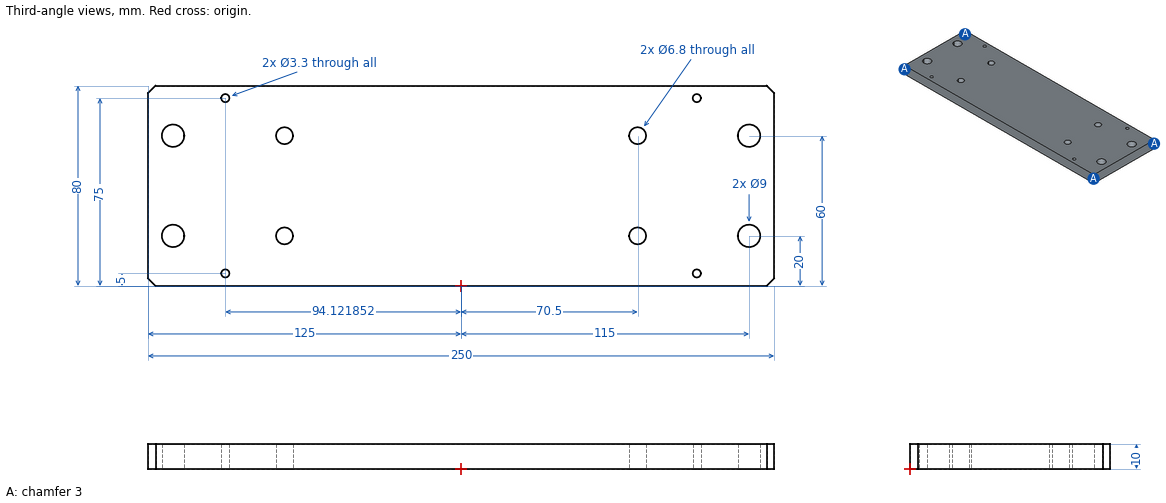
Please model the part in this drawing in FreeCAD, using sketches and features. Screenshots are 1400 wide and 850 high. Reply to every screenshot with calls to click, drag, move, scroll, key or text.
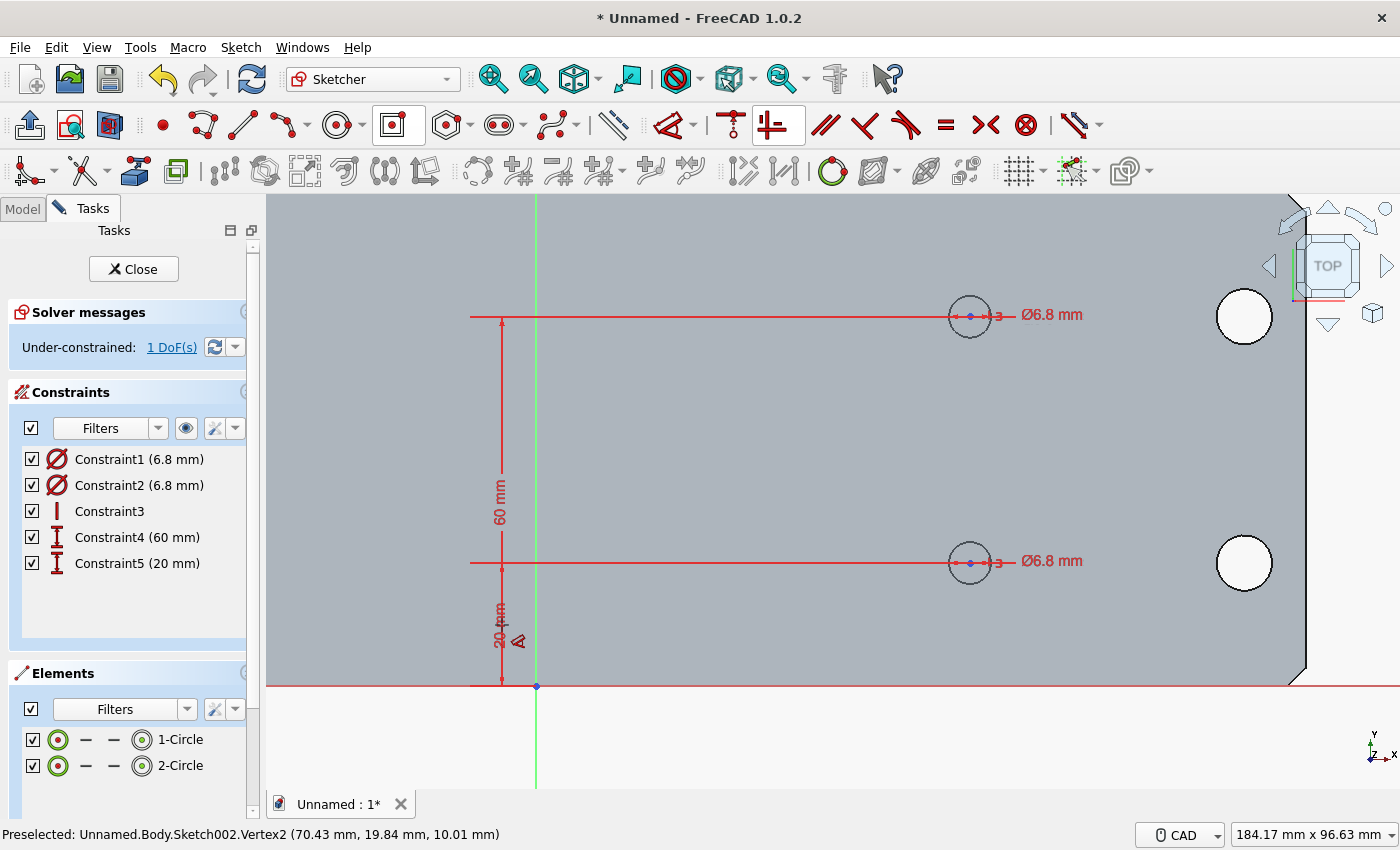
click(970, 317)
click(753, 720)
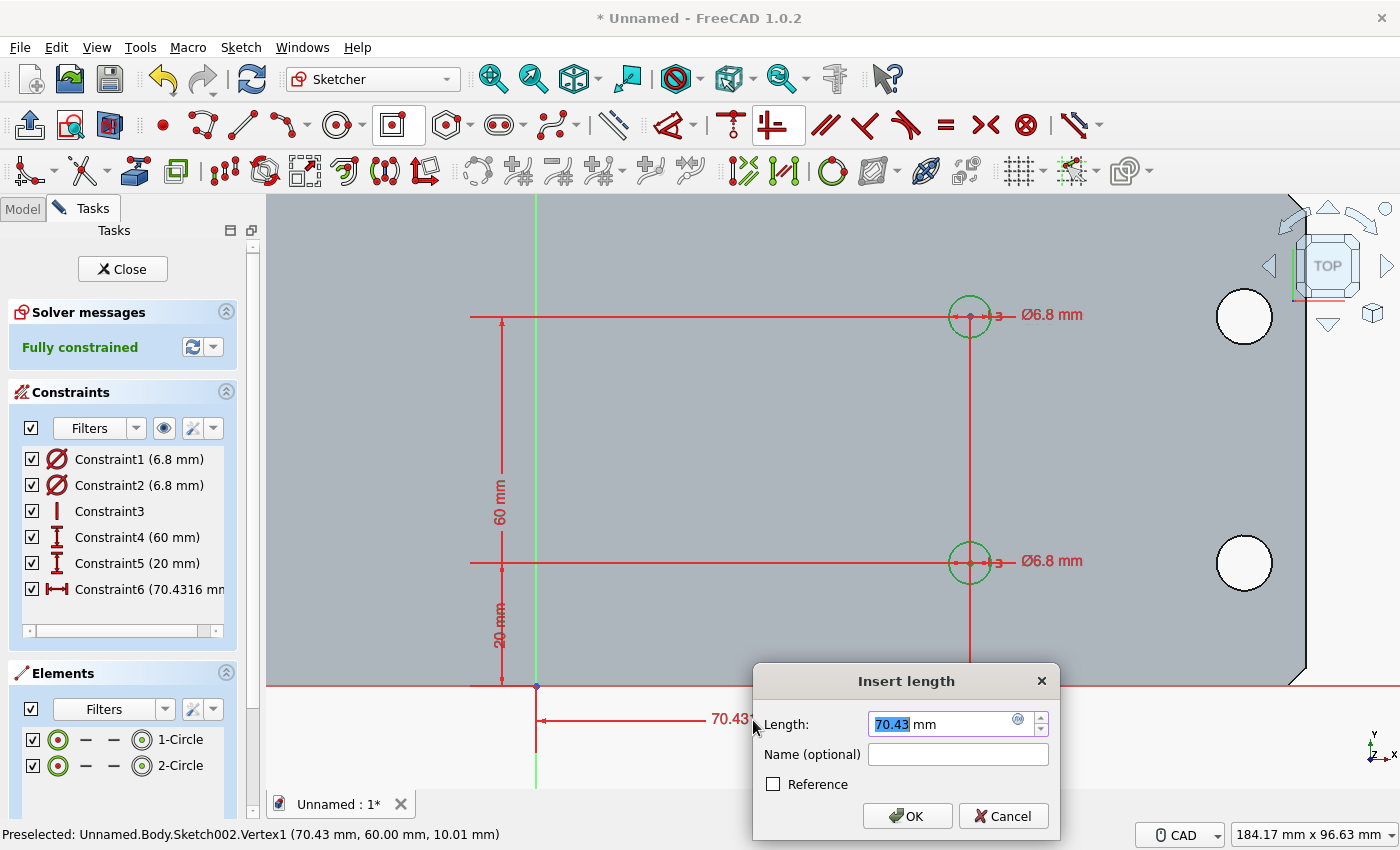
text(70.5)
key(Return)
key(Escape)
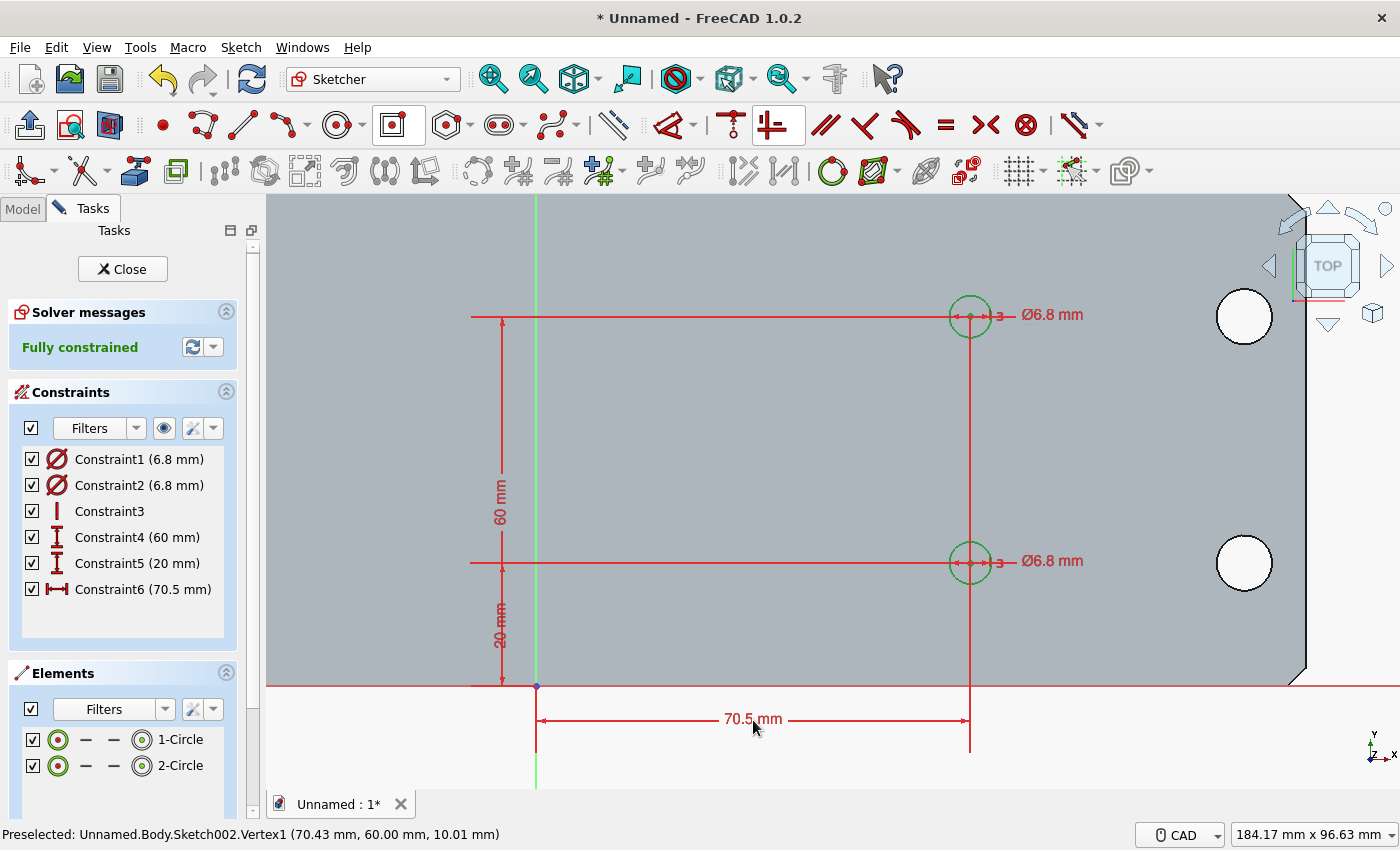
click(123, 269)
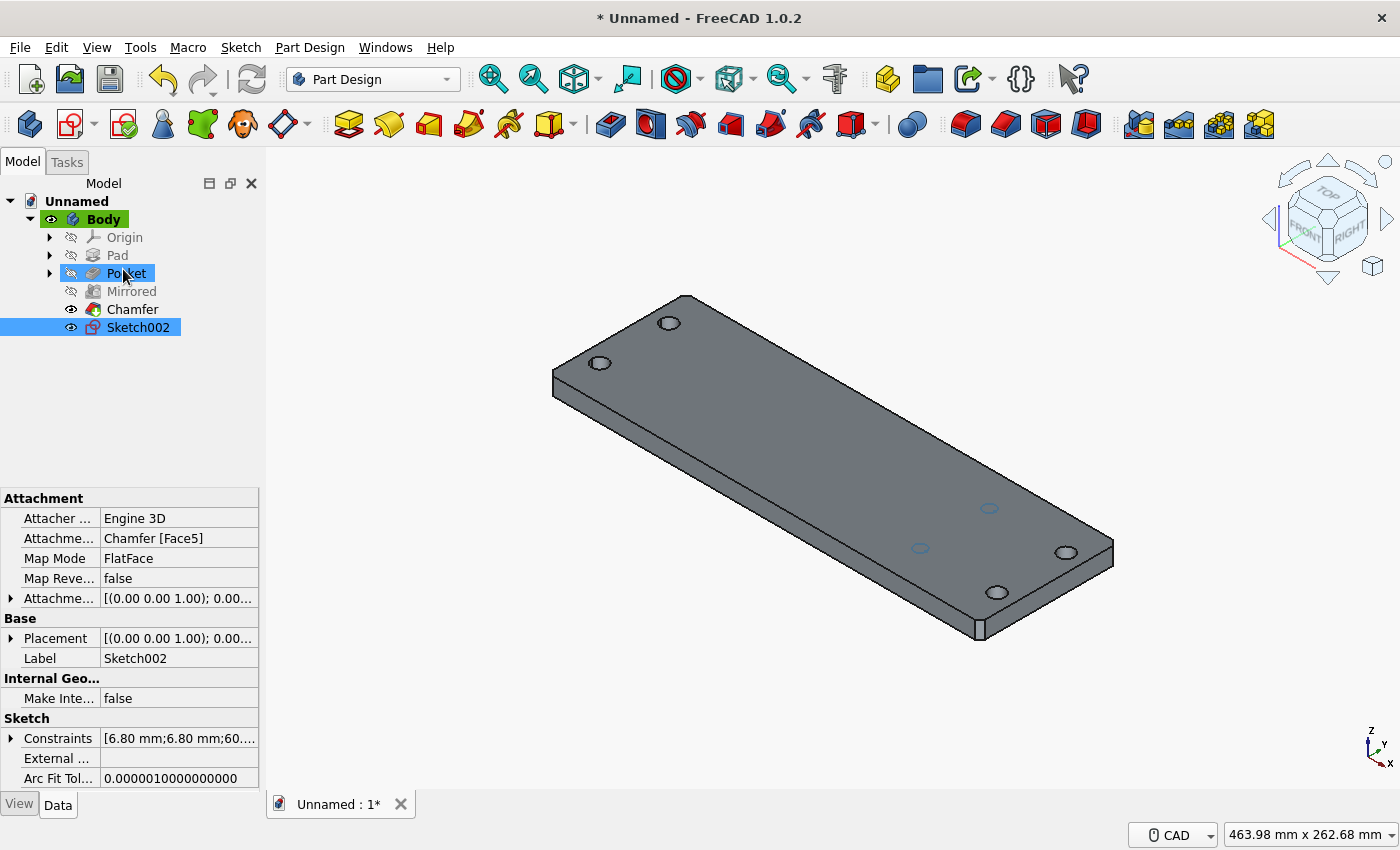
click(652, 124)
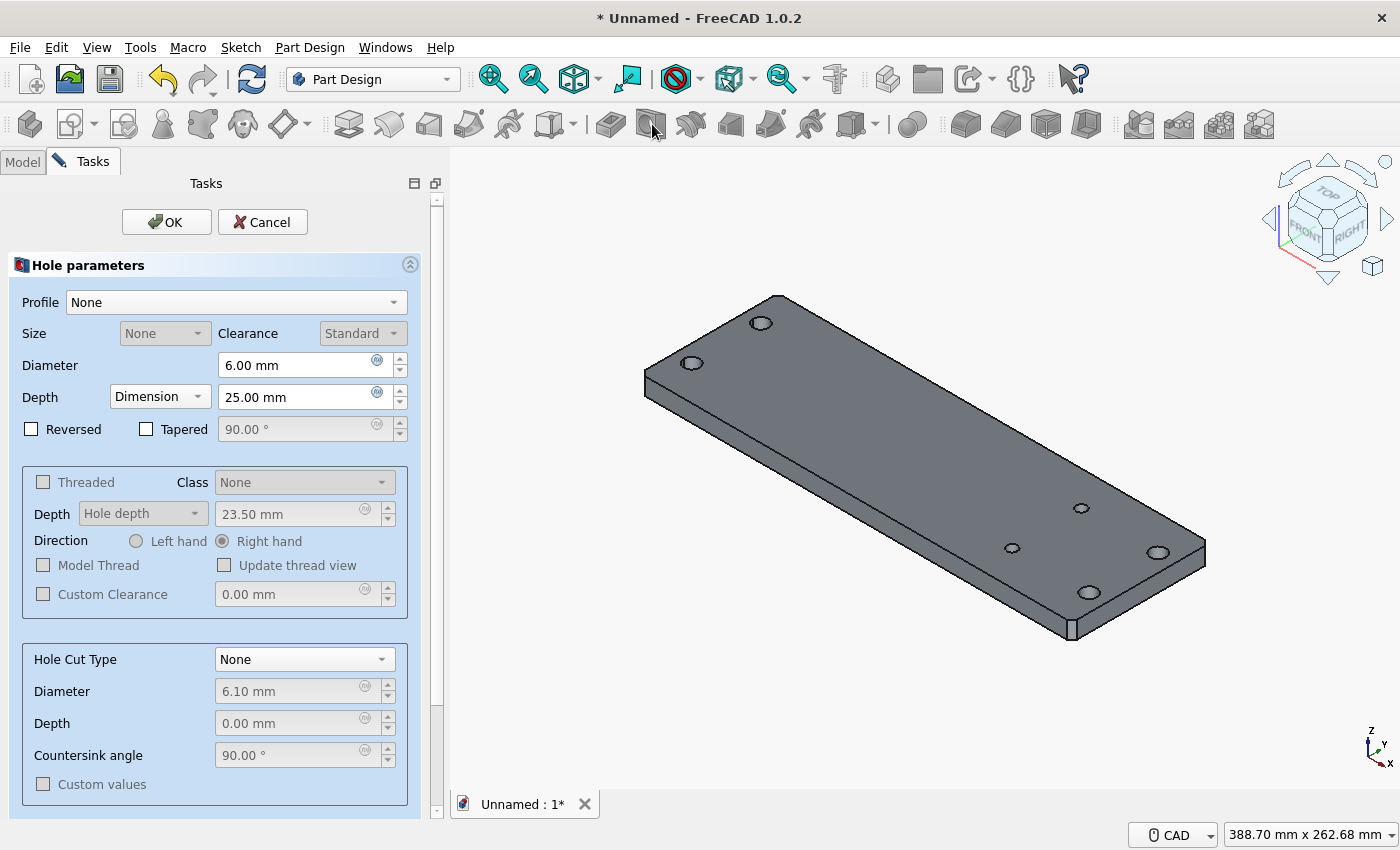
triple_click(305, 365)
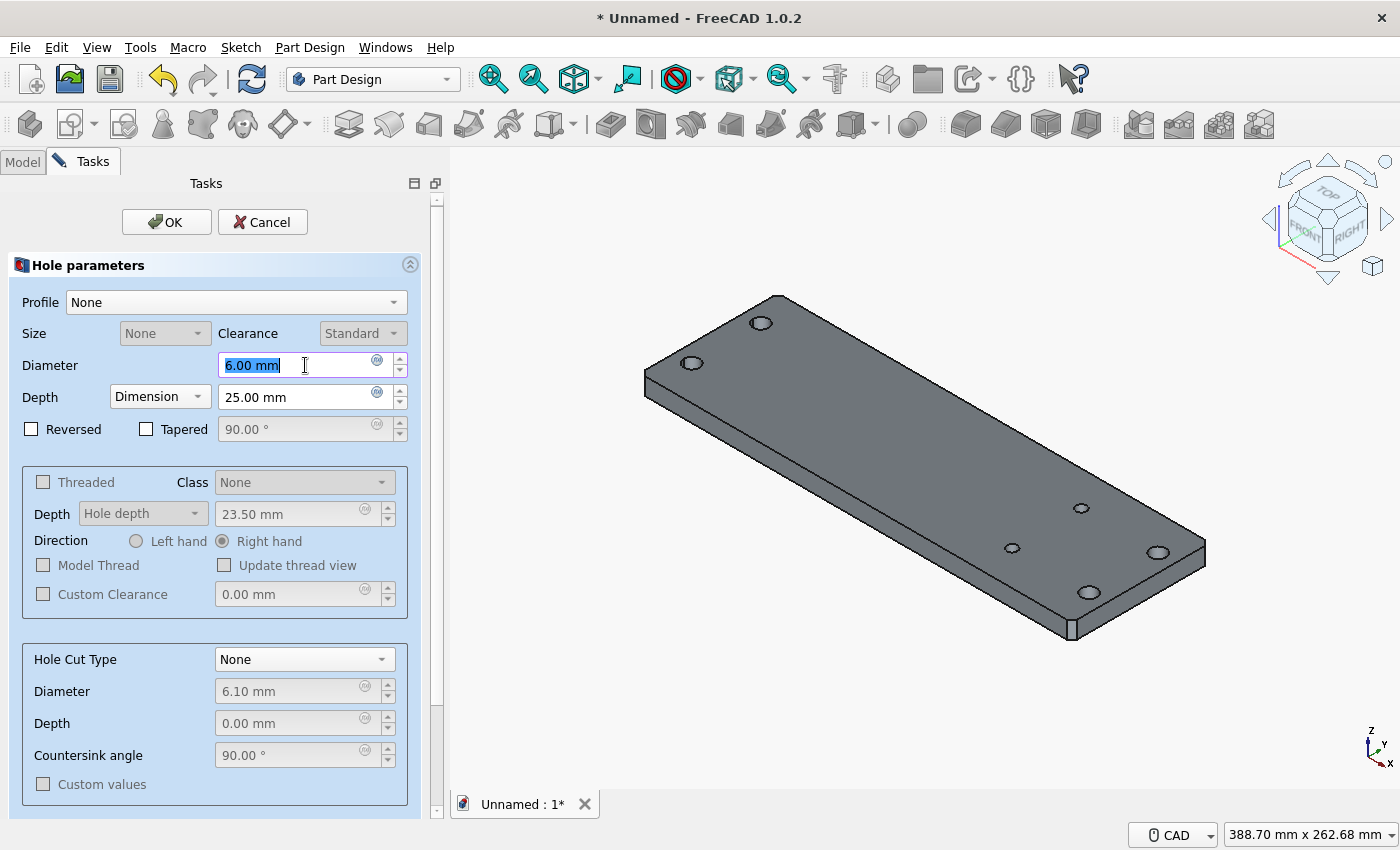
text(6.8)
key(Tab)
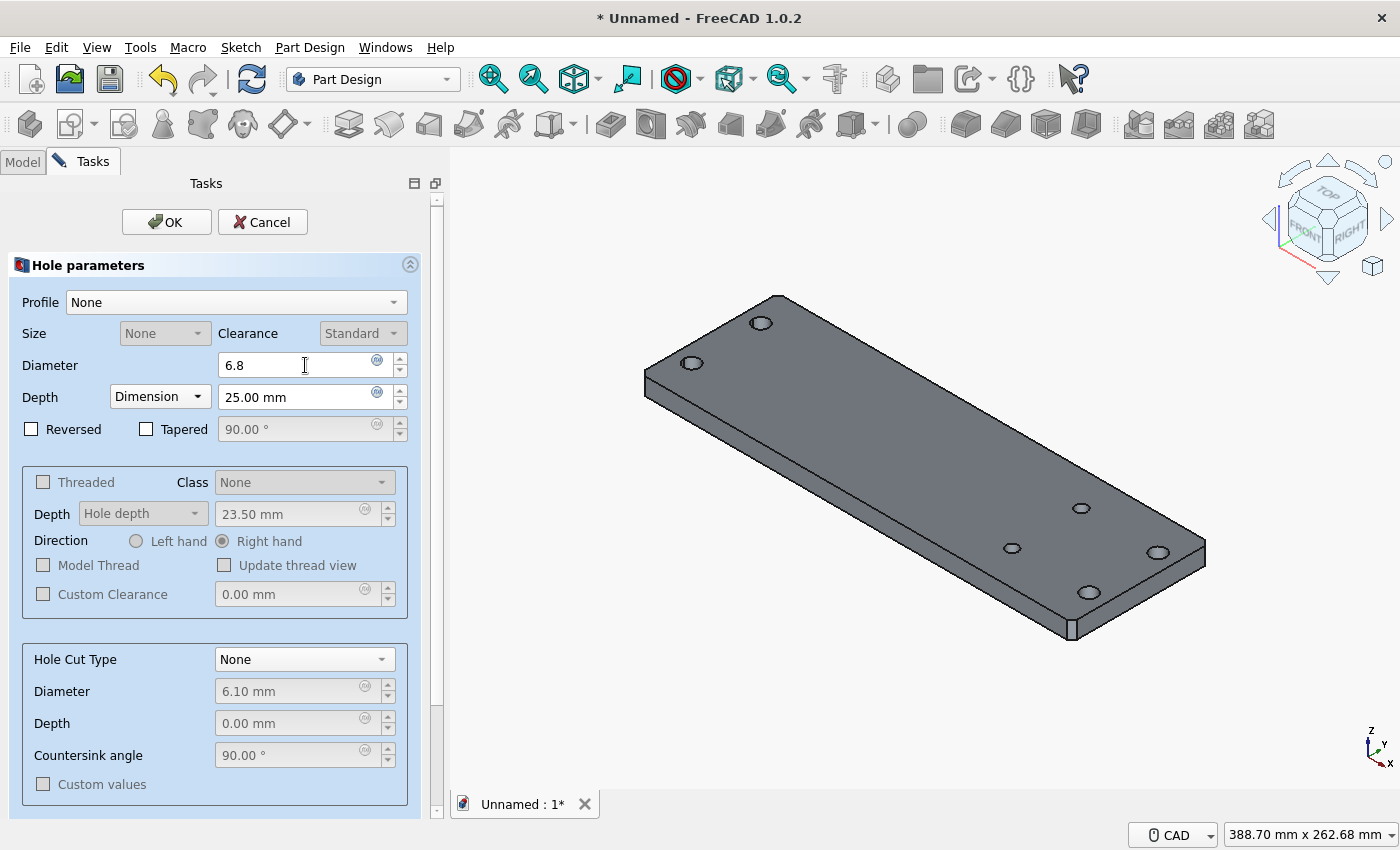
click(161, 396)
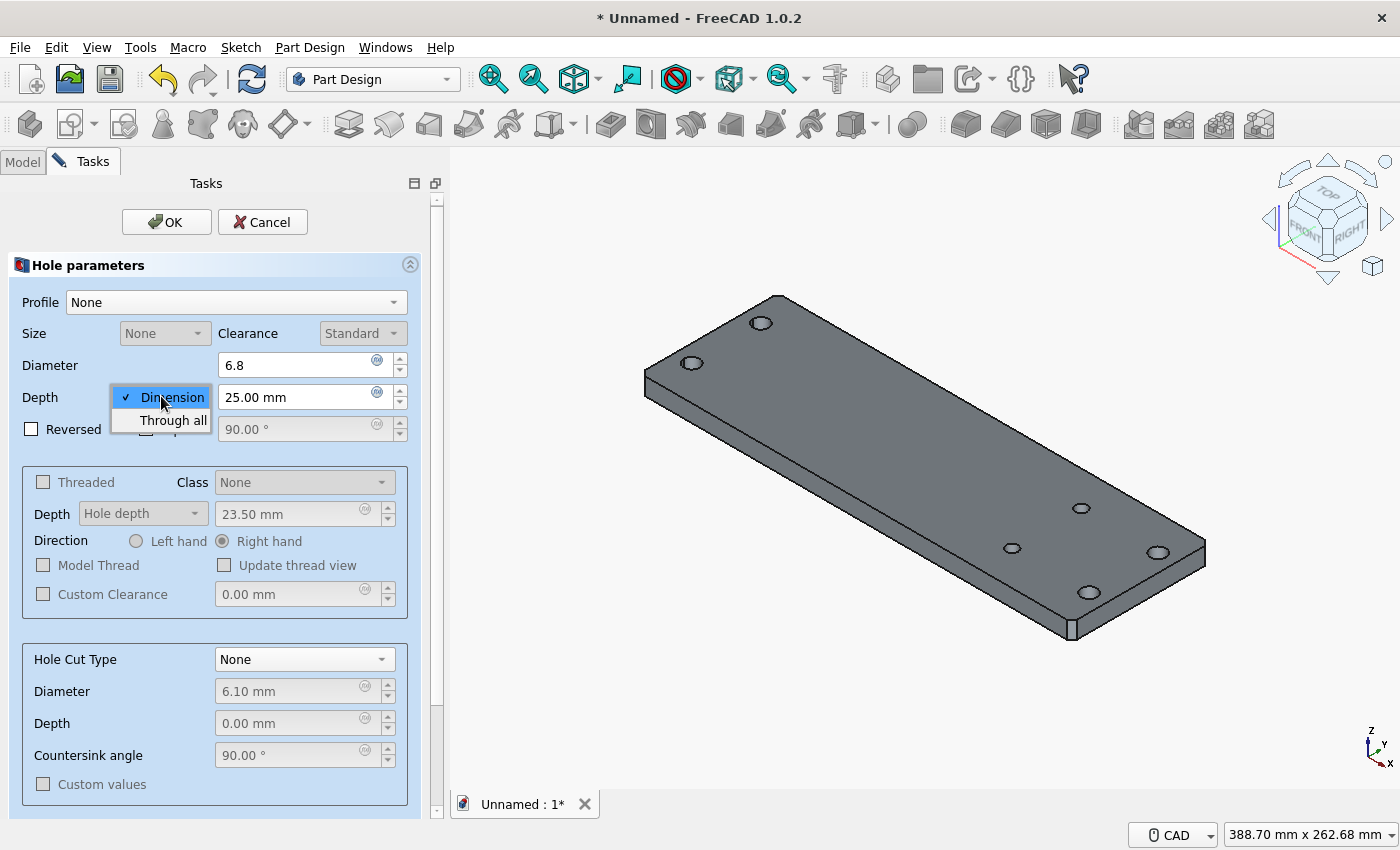
click(160, 420)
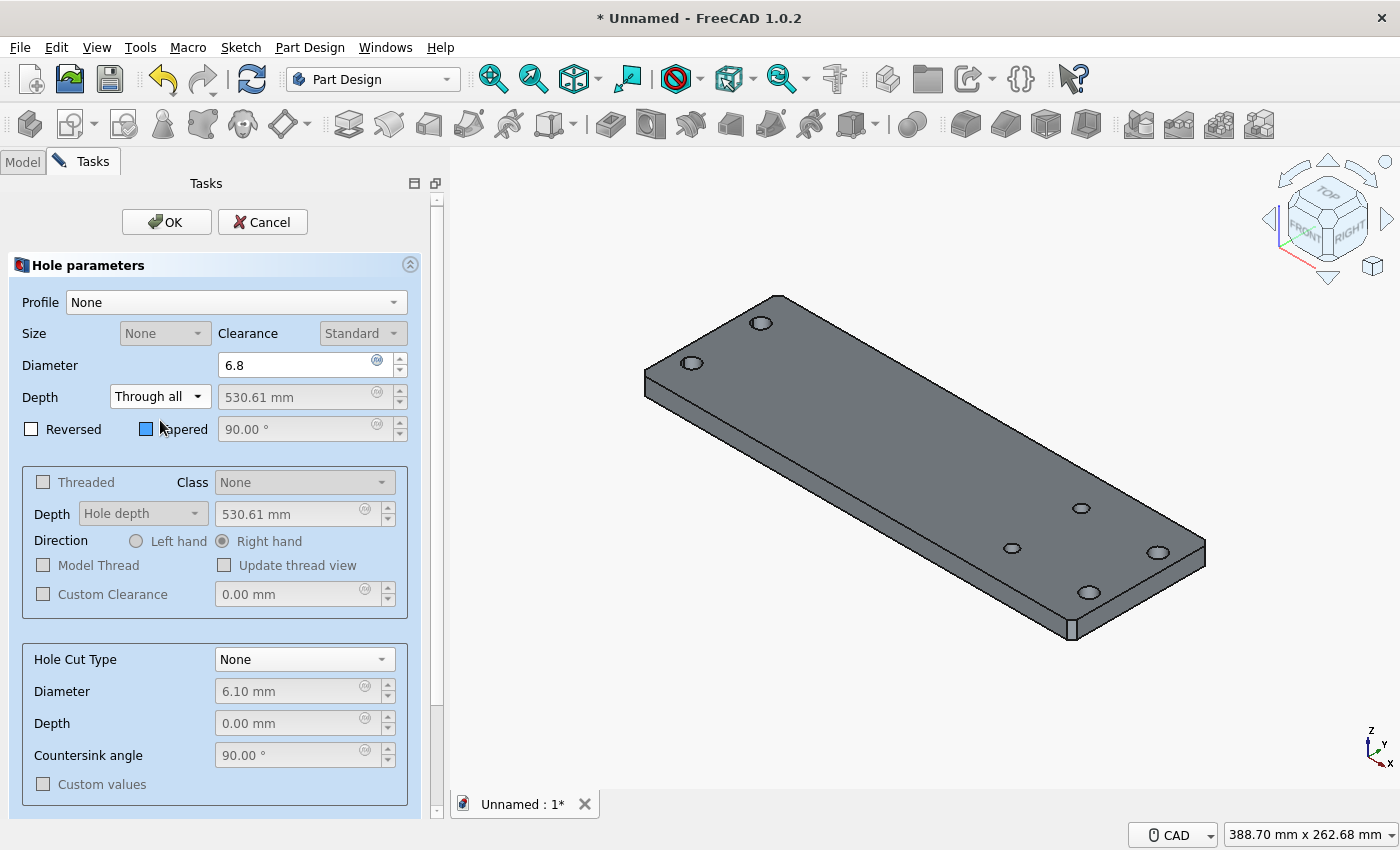
click(167, 222)